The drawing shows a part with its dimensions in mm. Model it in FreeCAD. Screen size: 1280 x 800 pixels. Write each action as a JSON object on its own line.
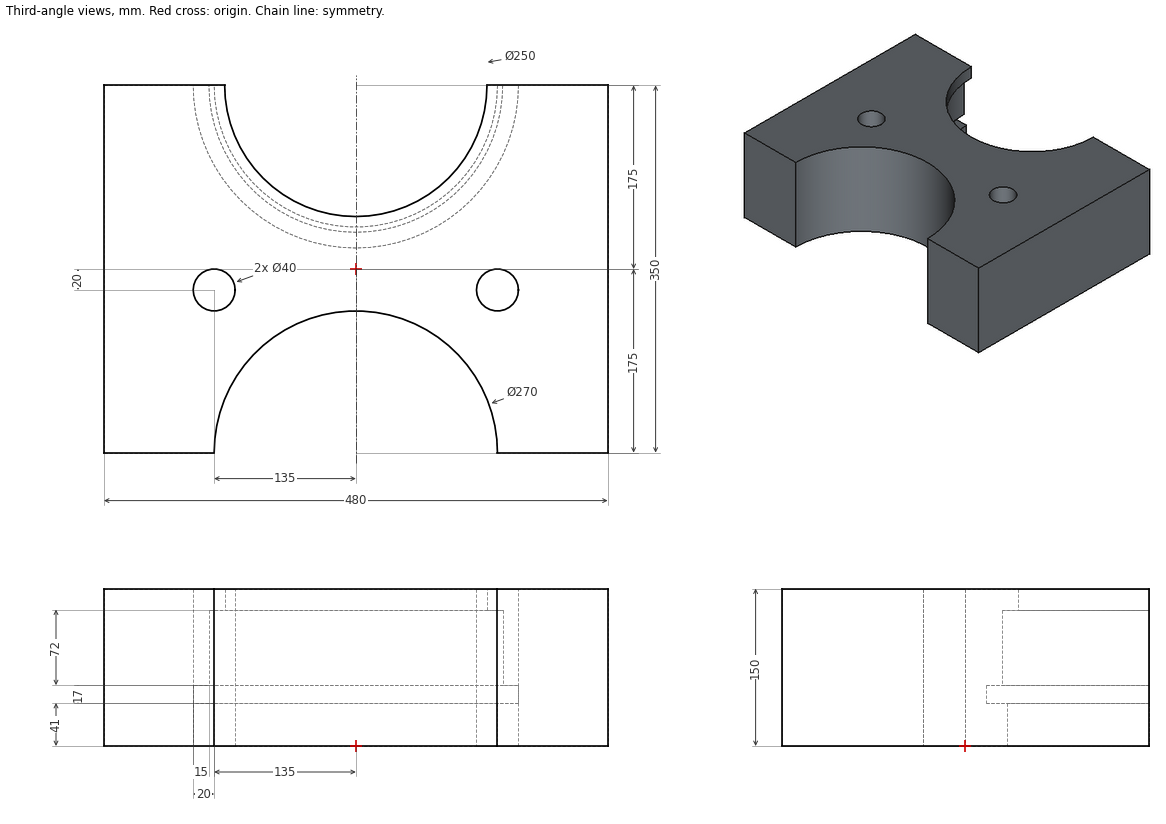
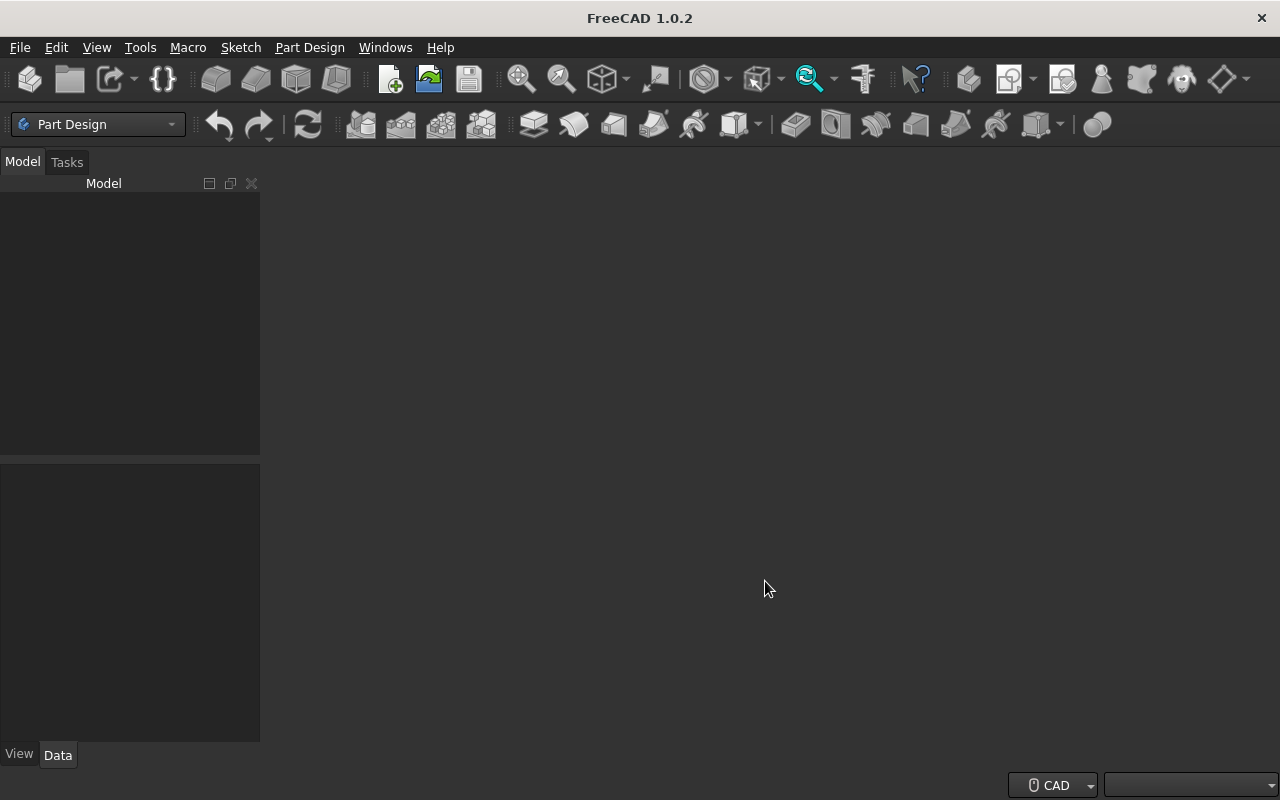
{"action": "key", "text": "ctrl+n"}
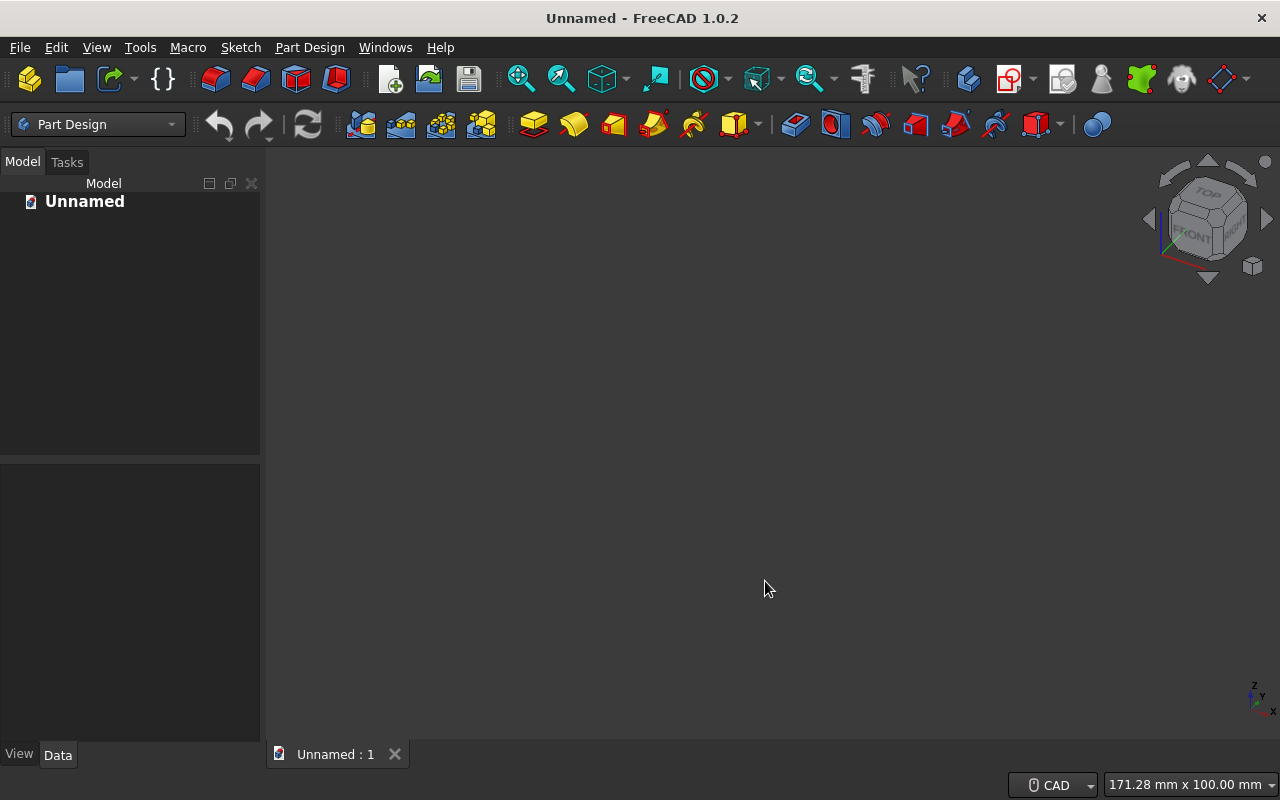
{"action": "left_click", "coordinate": [1010, 80]}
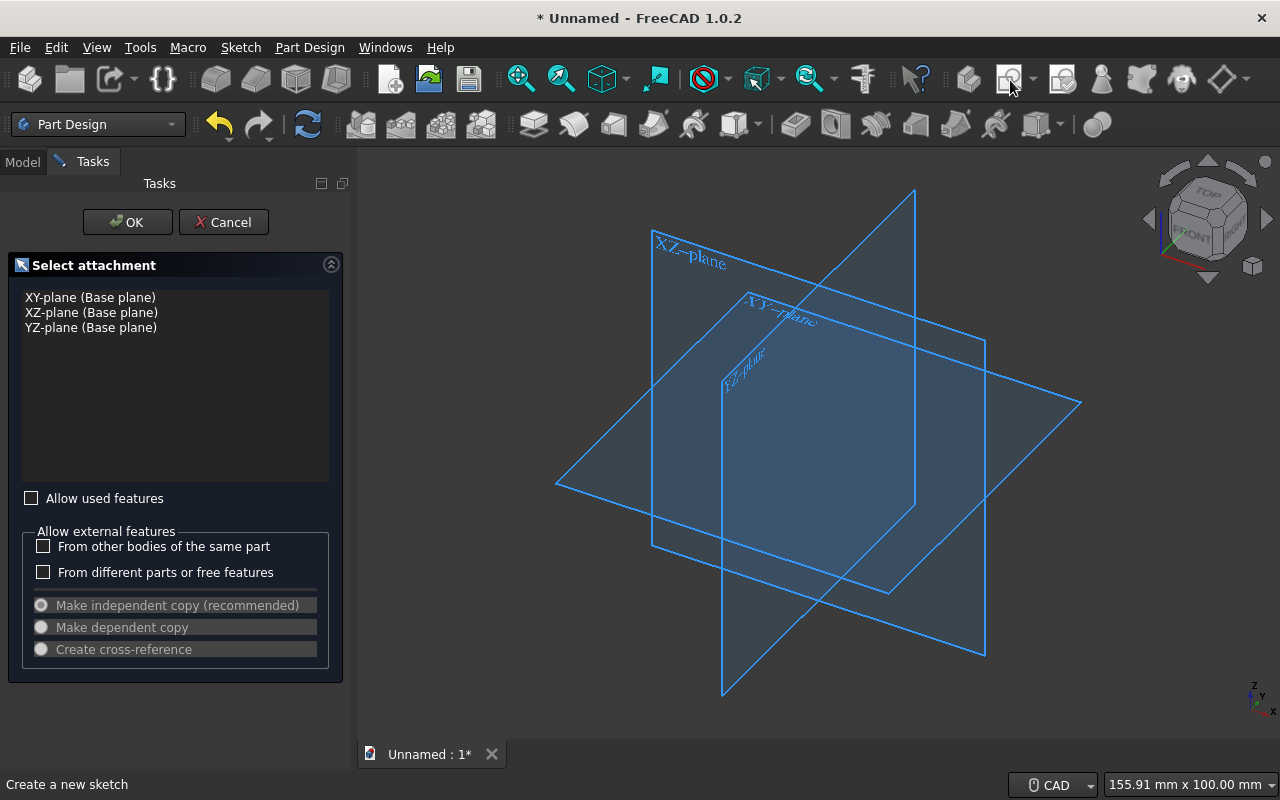
{"action": "left_click", "coordinate": [82, 298]}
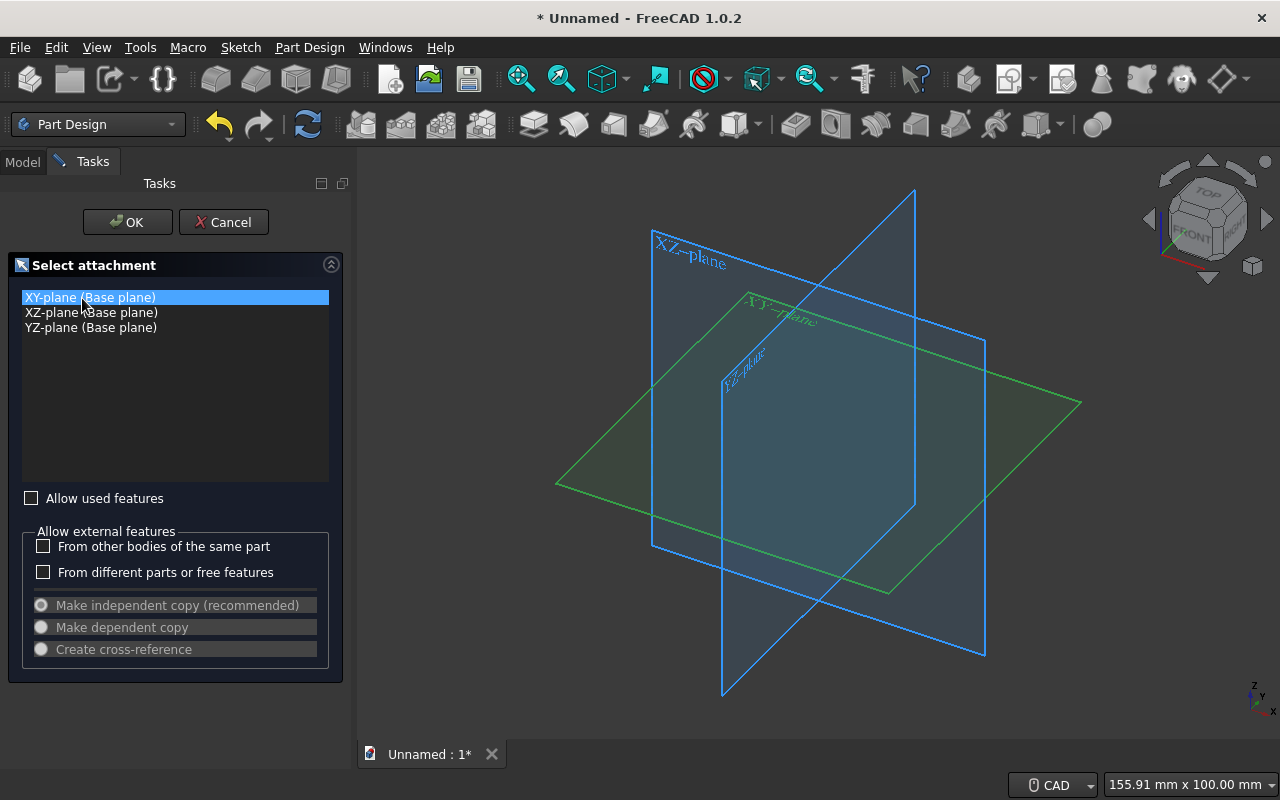
{"action": "left_click", "coordinate": [128, 222]}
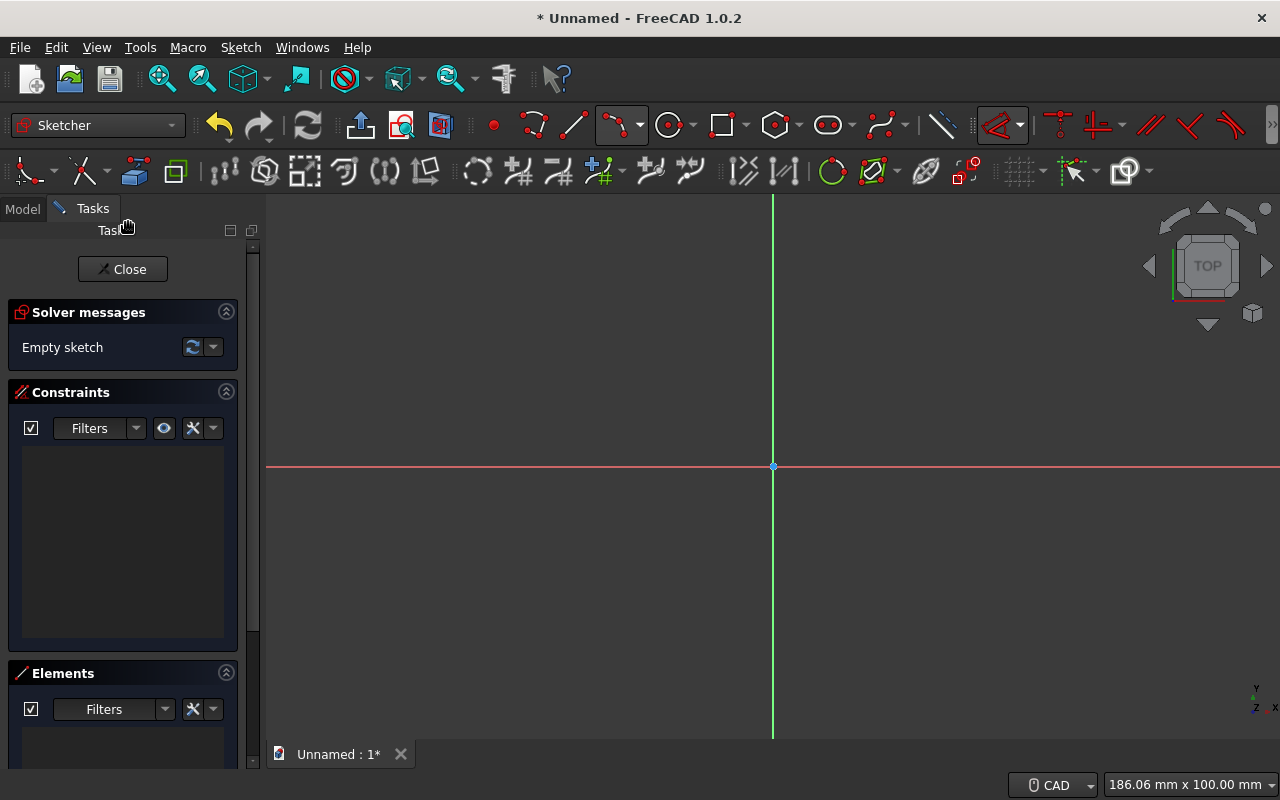
{"action": "scroll", "coordinate": [691, 466], "scroll_direction": "down", "scroll_amount": 9}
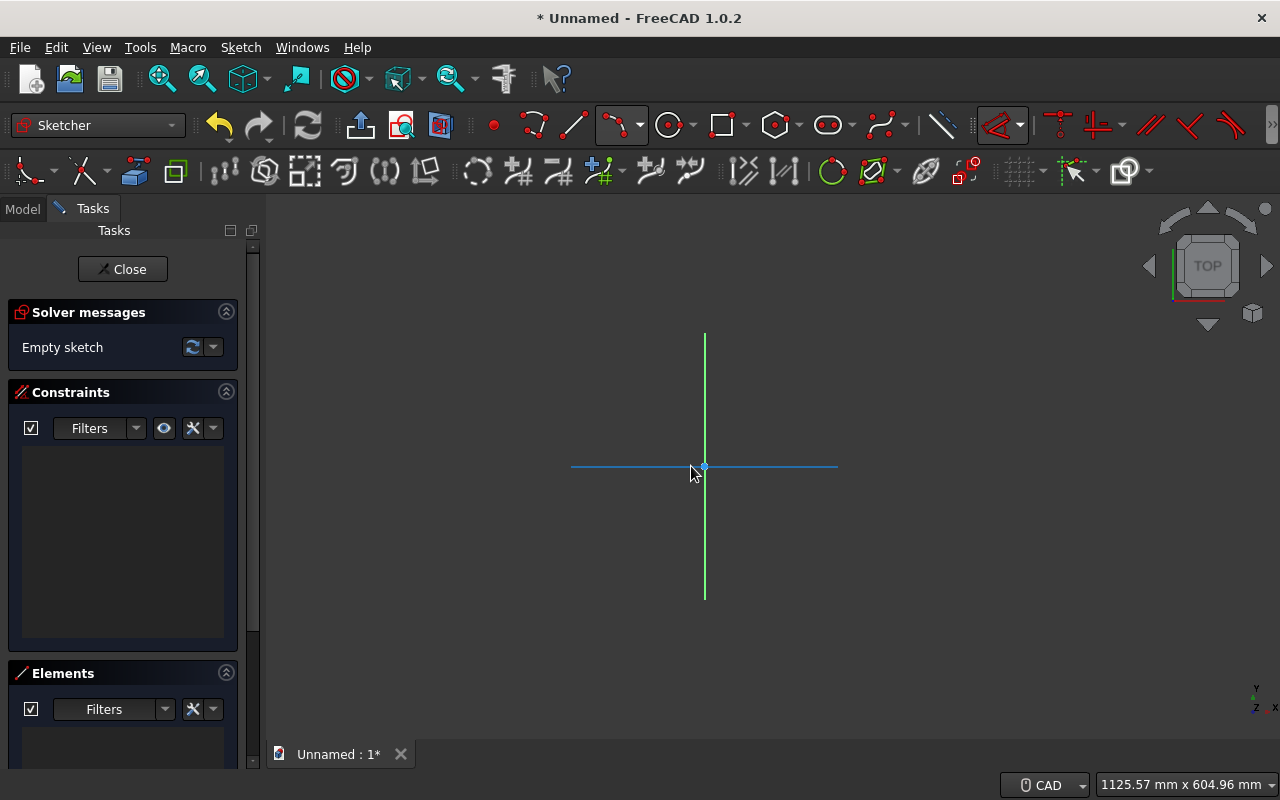
{"action": "key", "text": "g v"}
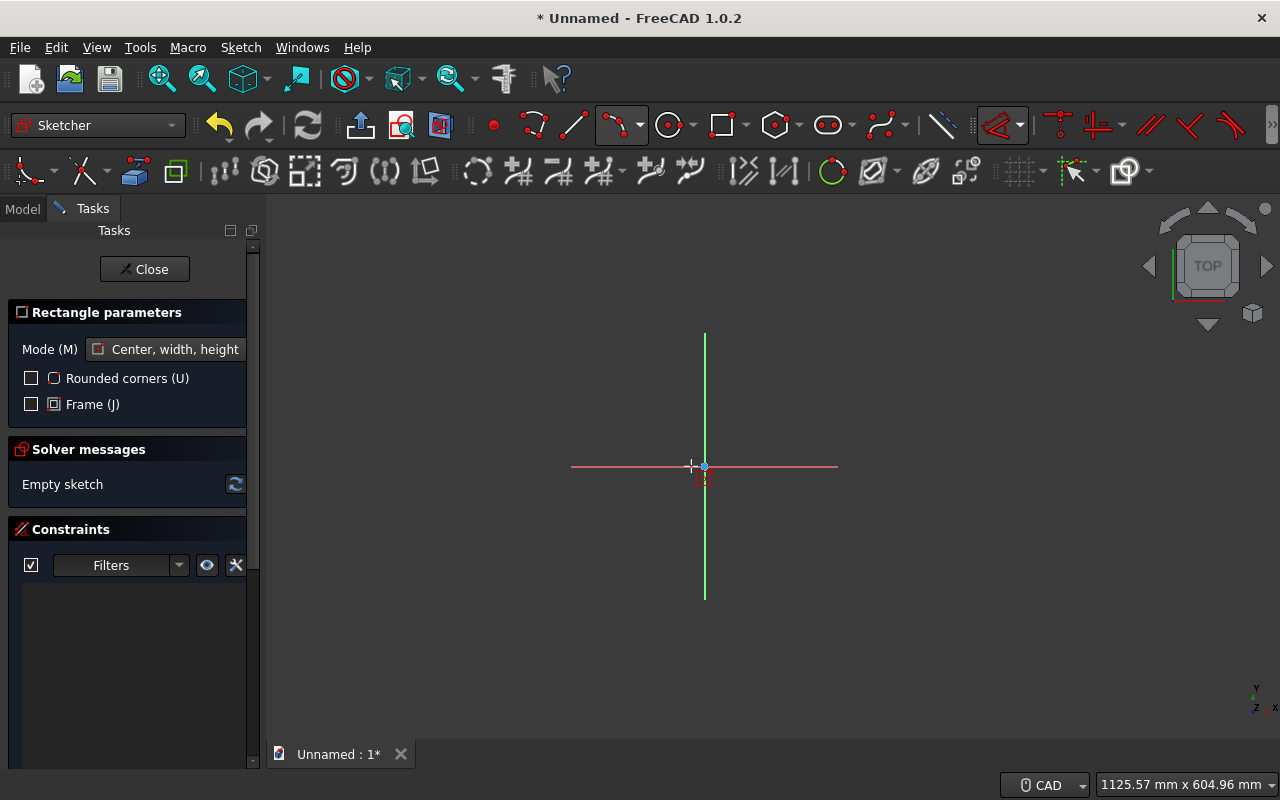
{"action": "left_click", "coordinate": [705, 466]}
{"action": "mouse_move", "coordinate": [921, 309]}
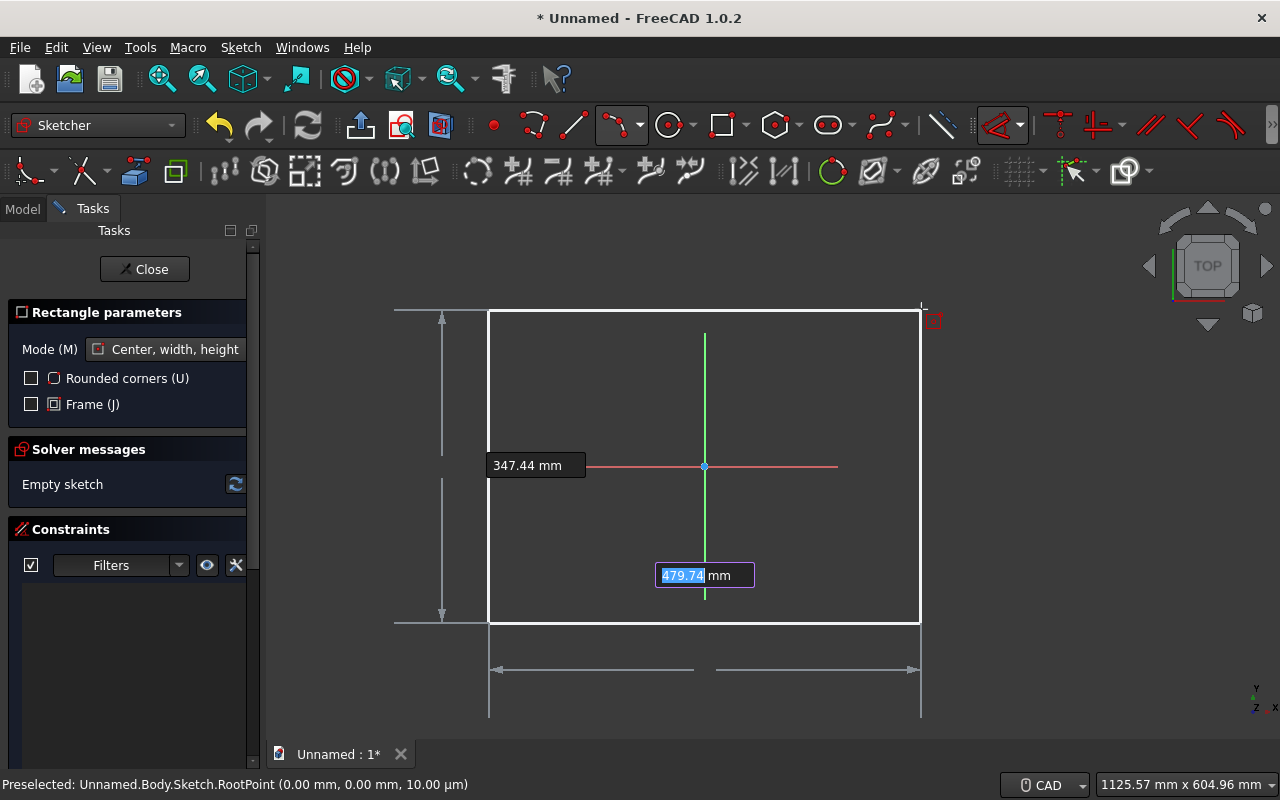
{"action": "type", "text": "480"}
{"action": "key", "text": "Tab"}
{"action": "type", "text": "350"}
{"action": "key", "text": "Return"}
{"action": "key", "text": "Escape"}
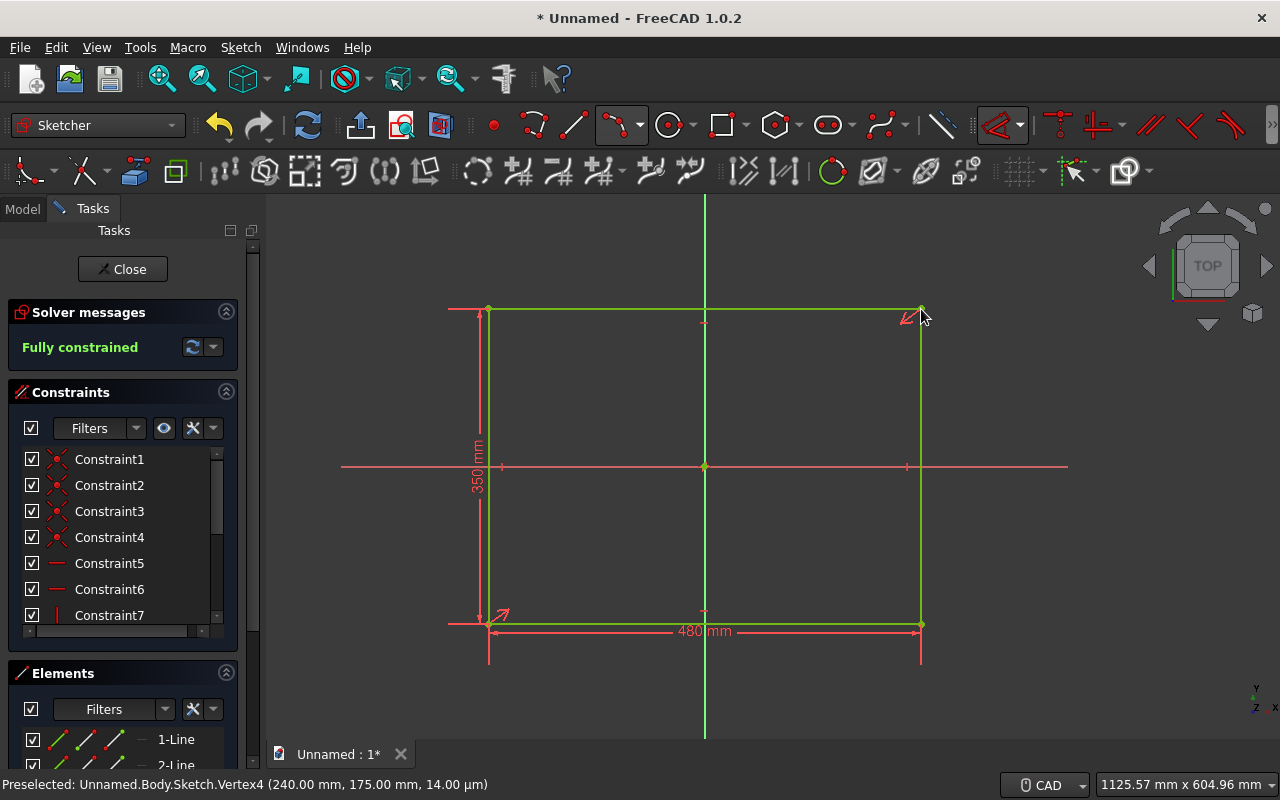
{"action": "left_click", "coordinate": [123, 269]}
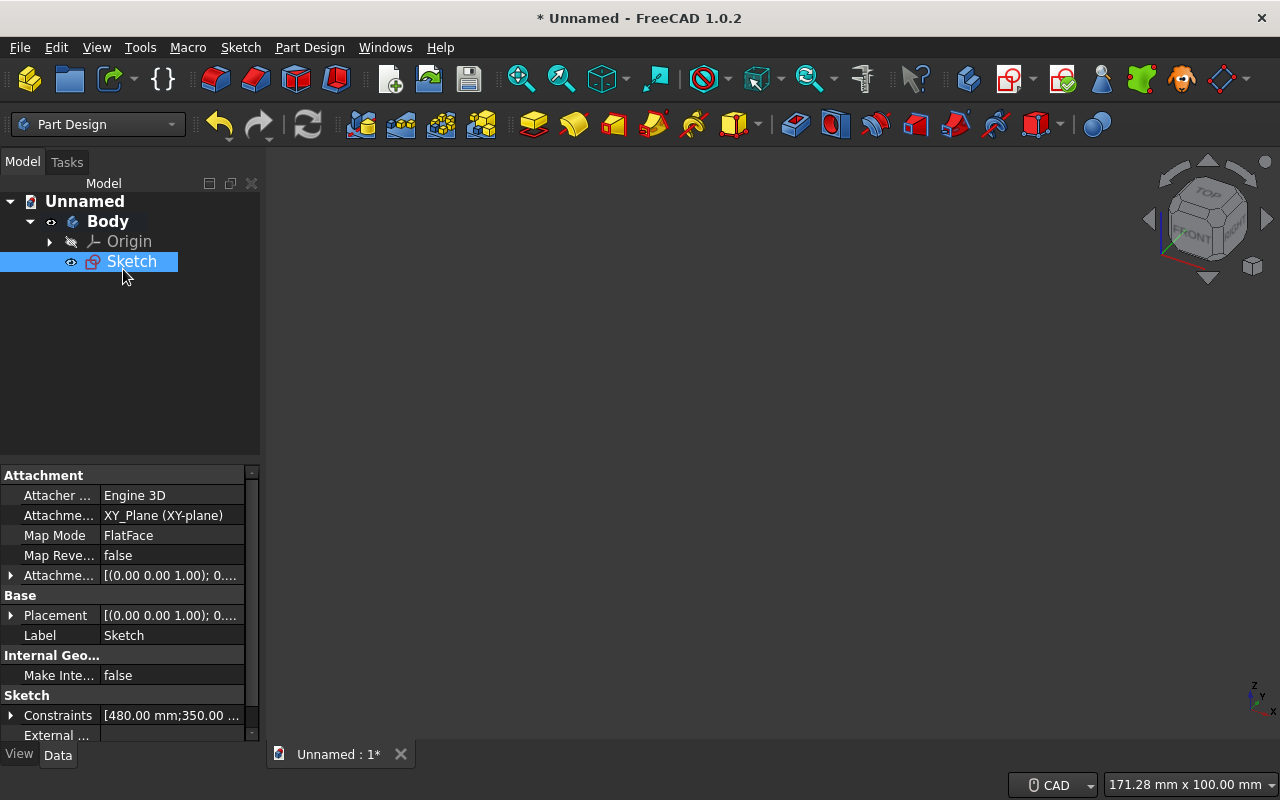
{"action": "left_click", "coordinate": [534, 124]}